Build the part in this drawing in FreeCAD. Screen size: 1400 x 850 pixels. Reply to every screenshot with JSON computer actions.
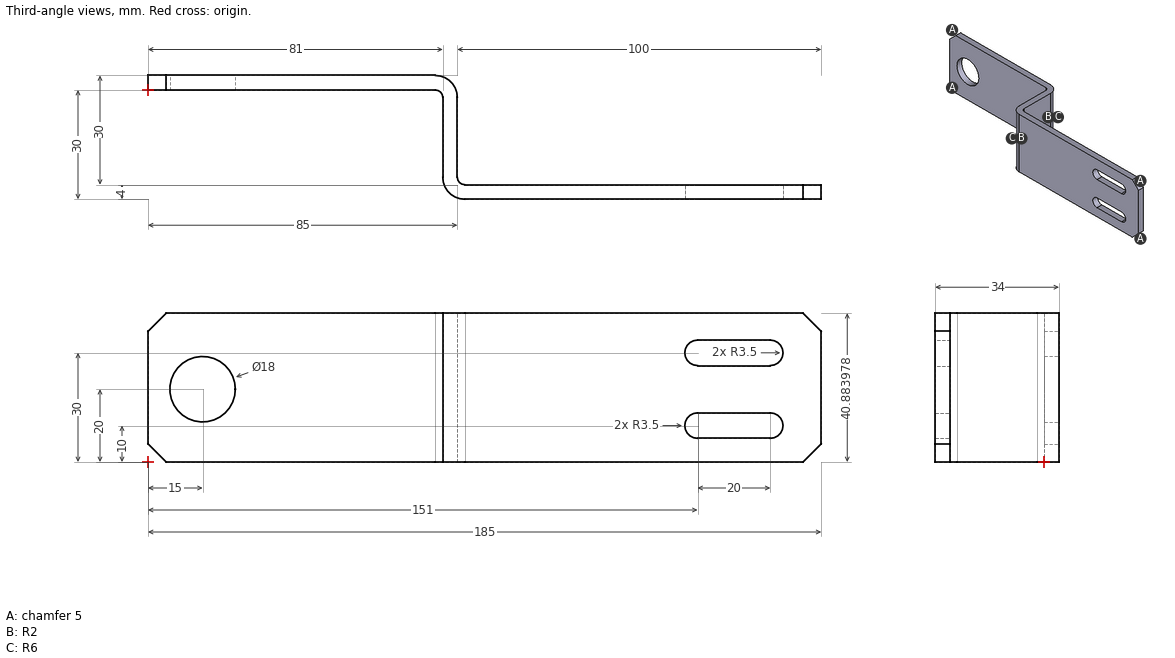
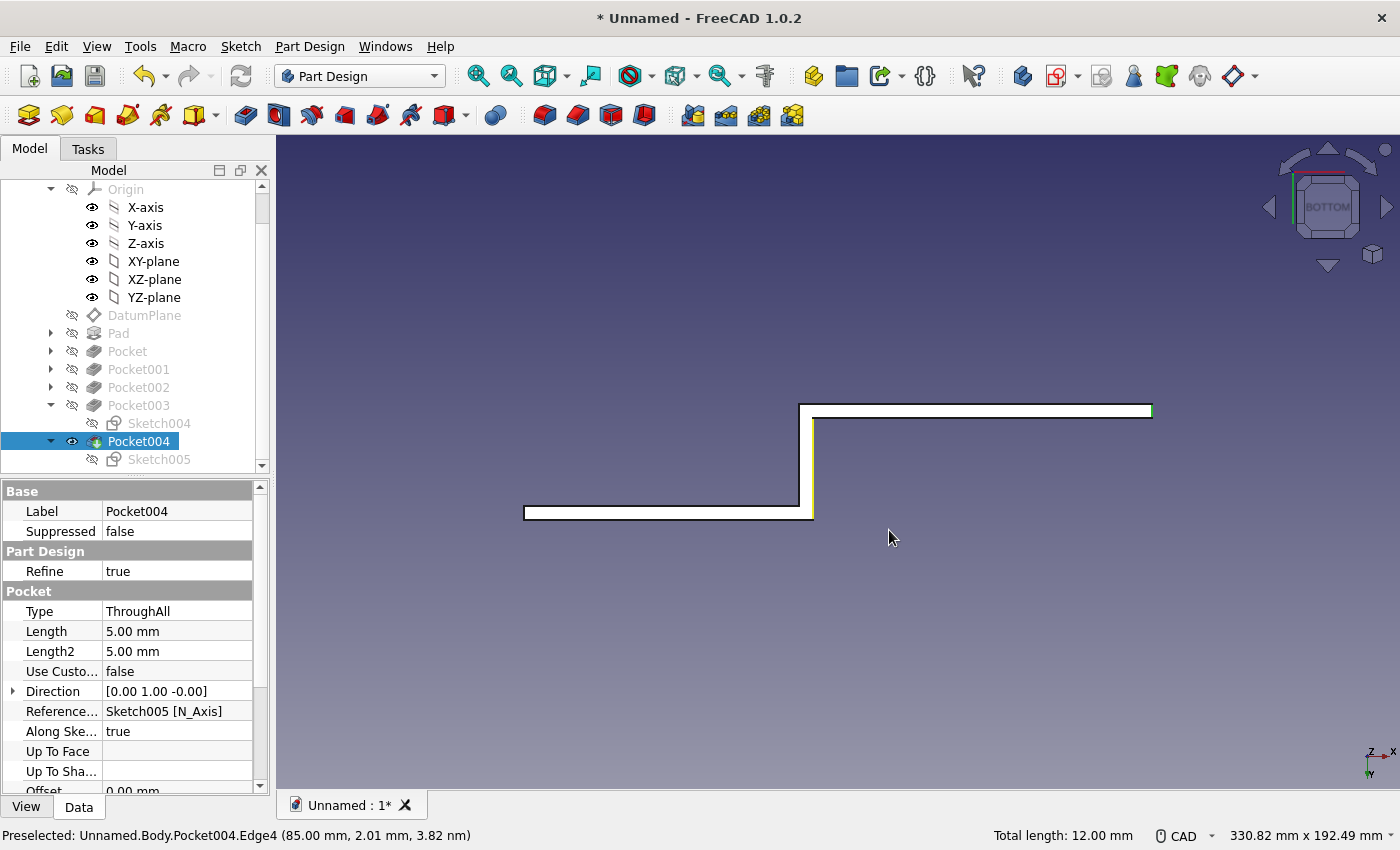
{"action": "scroll", "coordinate": [524, 512], "scroll_direction": "up", "scroll_amount": 6}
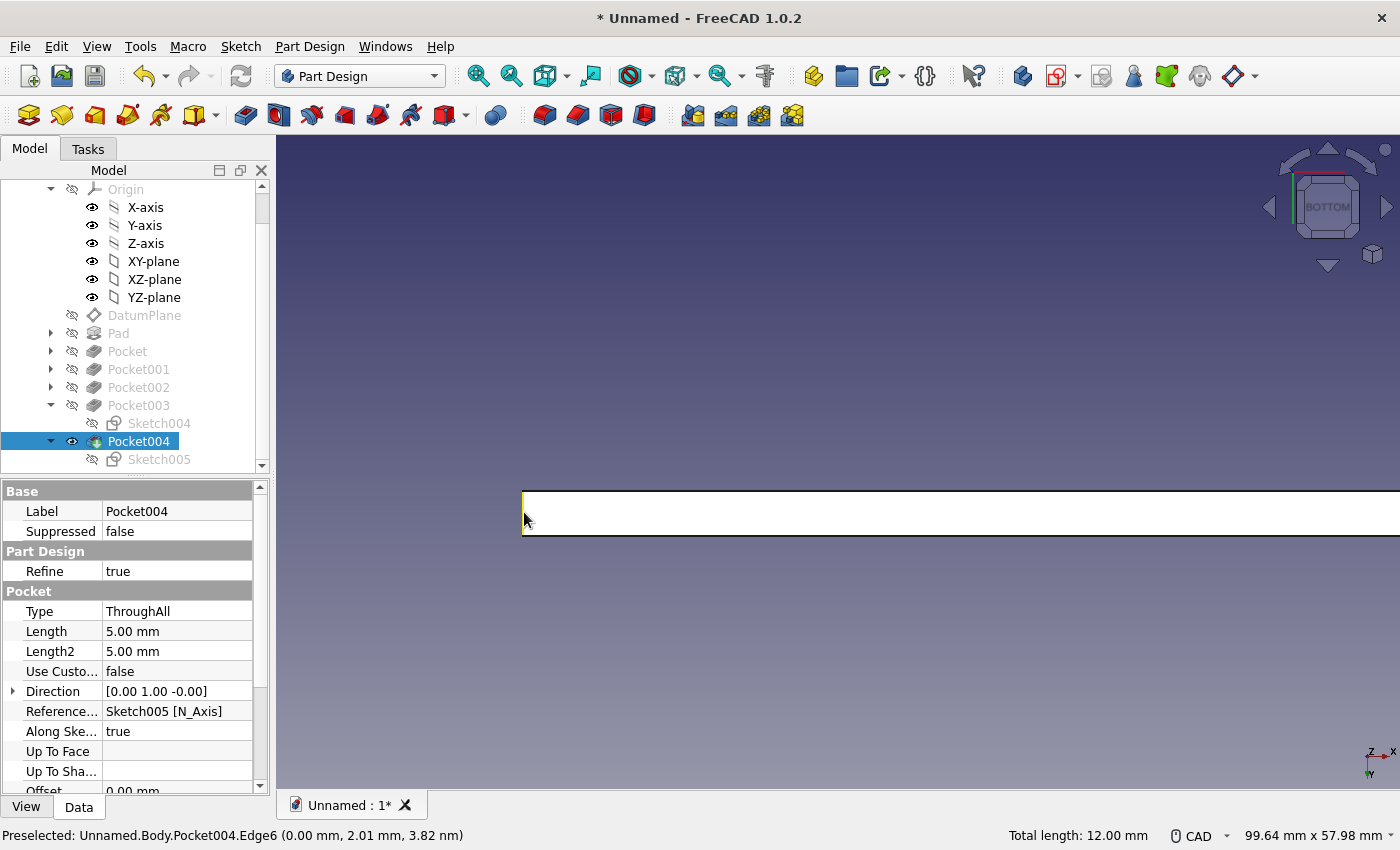
{"action": "left_click", "coordinate": [479, 76]}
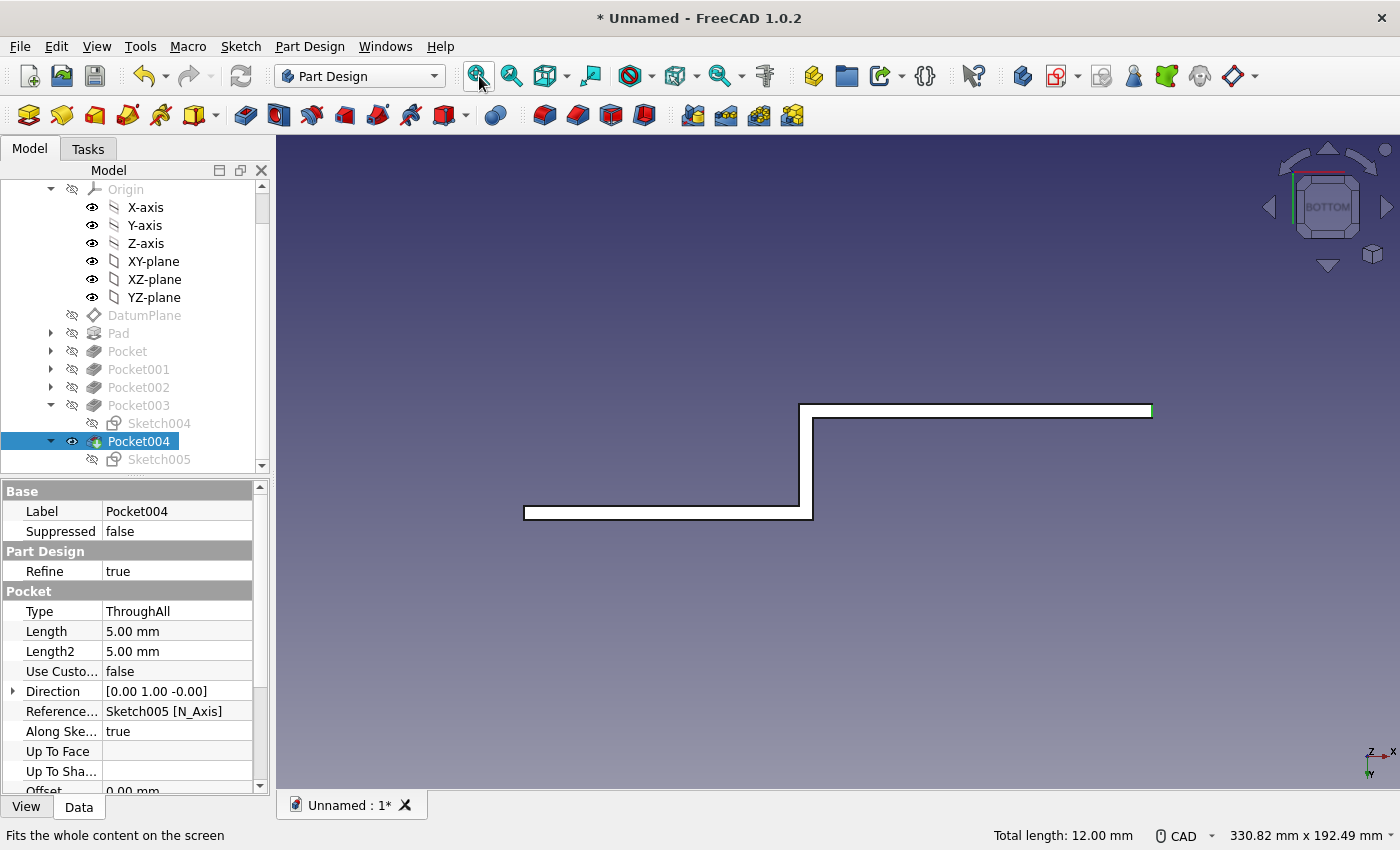
{"action": "key", "text": "4"}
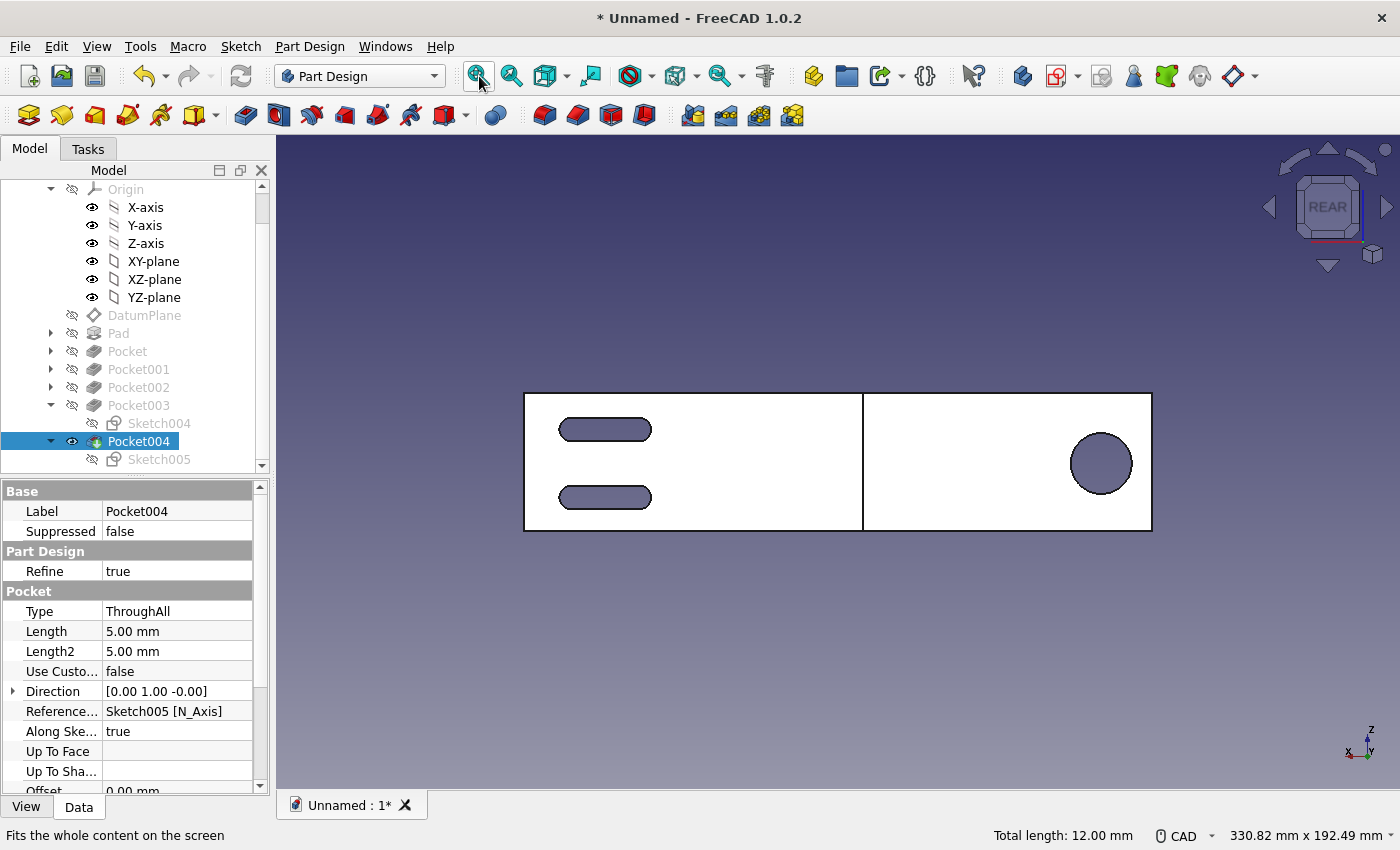
{"action": "scroll", "coordinate": [1152, 530], "scroll_direction": "up", "scroll_amount": 6}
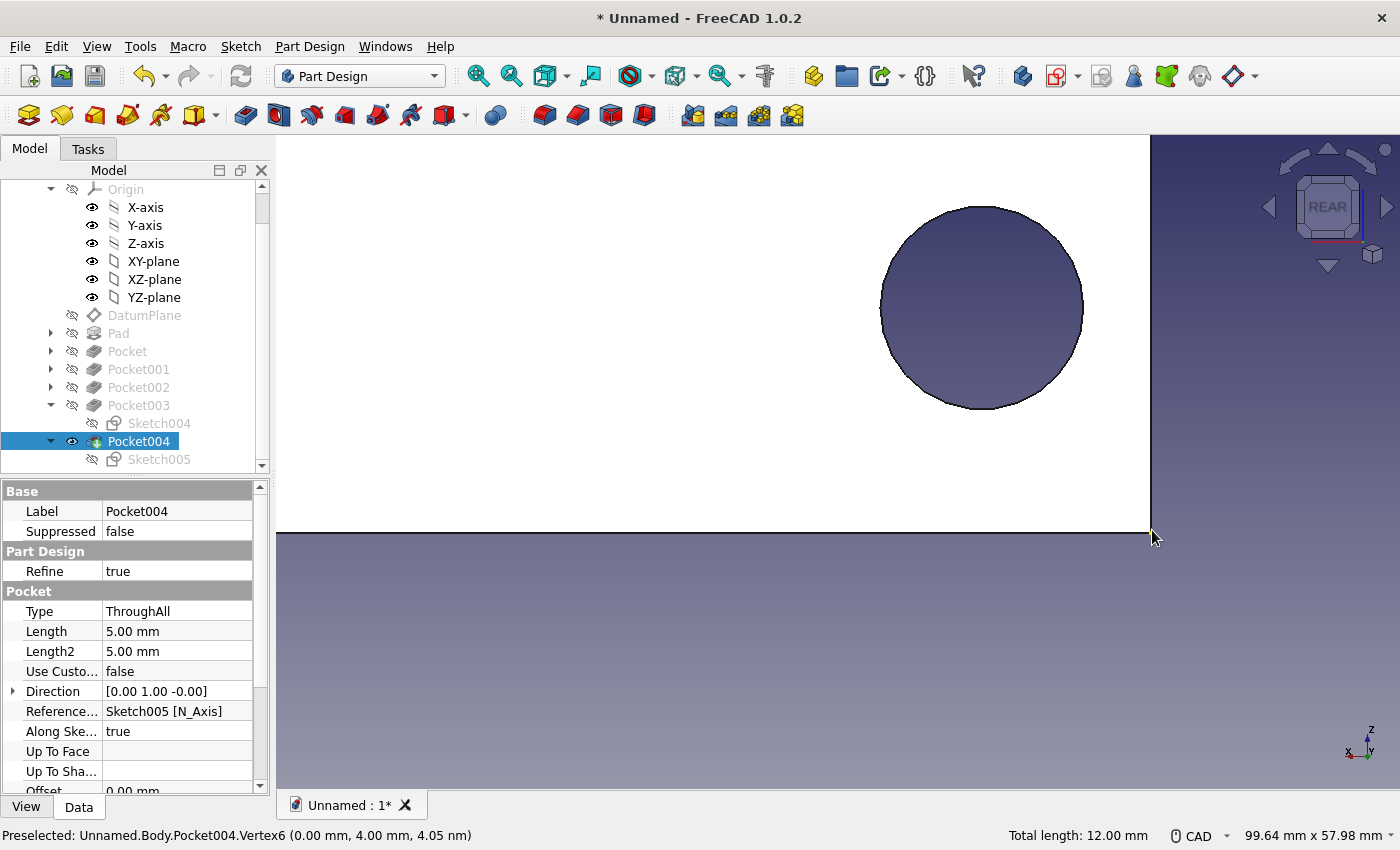
{"action": "key", "text": "v f"}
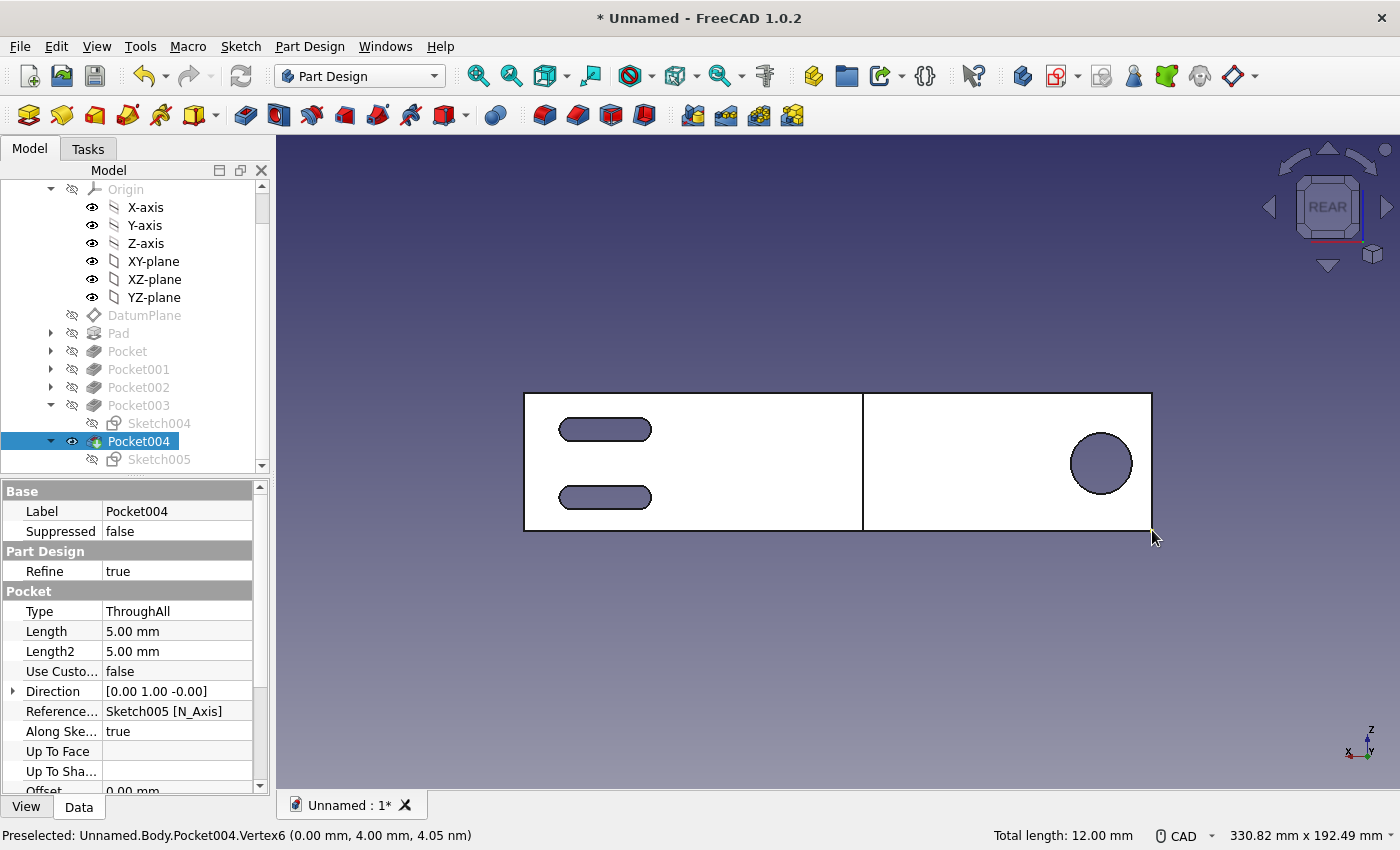
{"action": "key", "text": "6"}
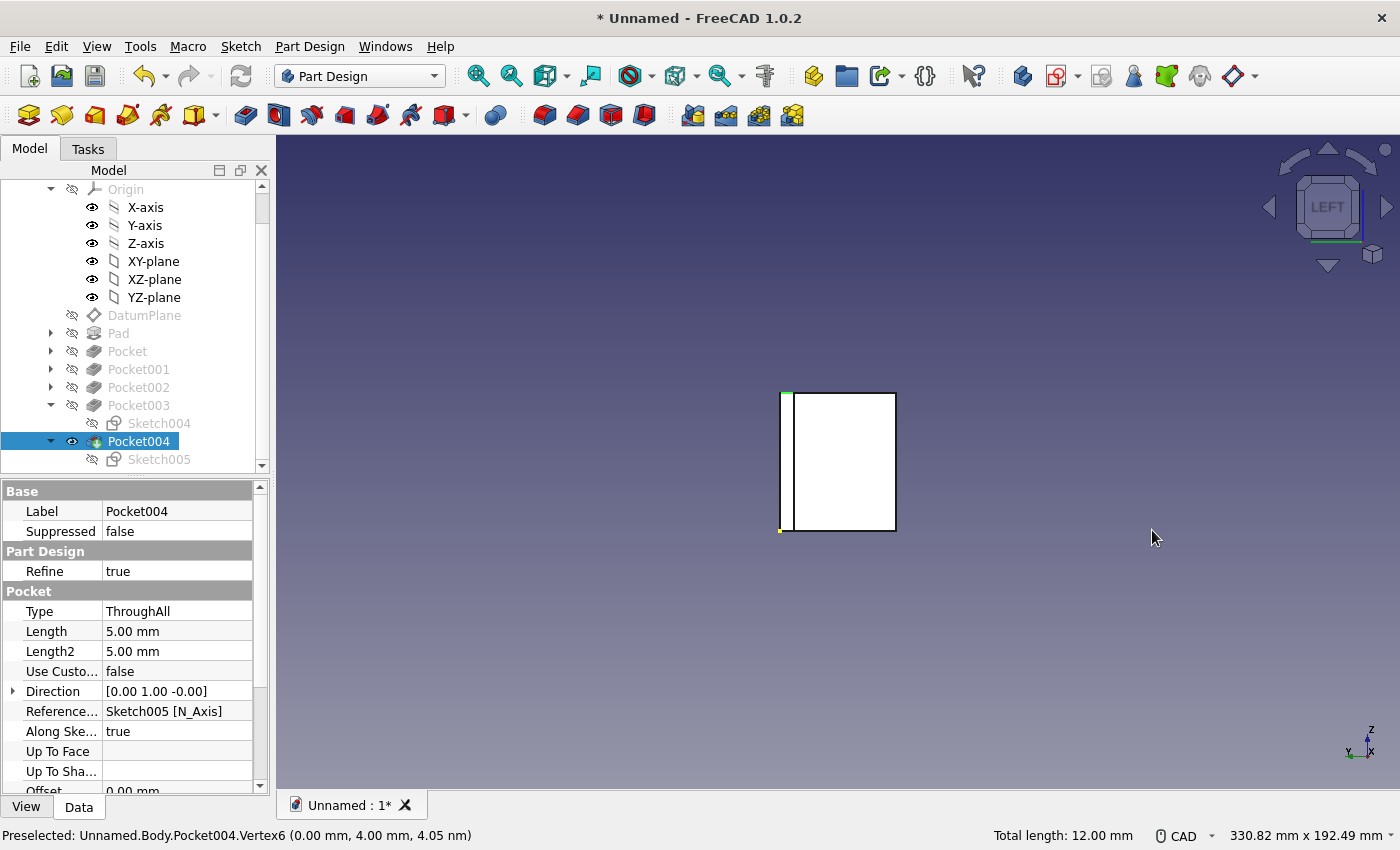
{"action": "key", "text": "v f"}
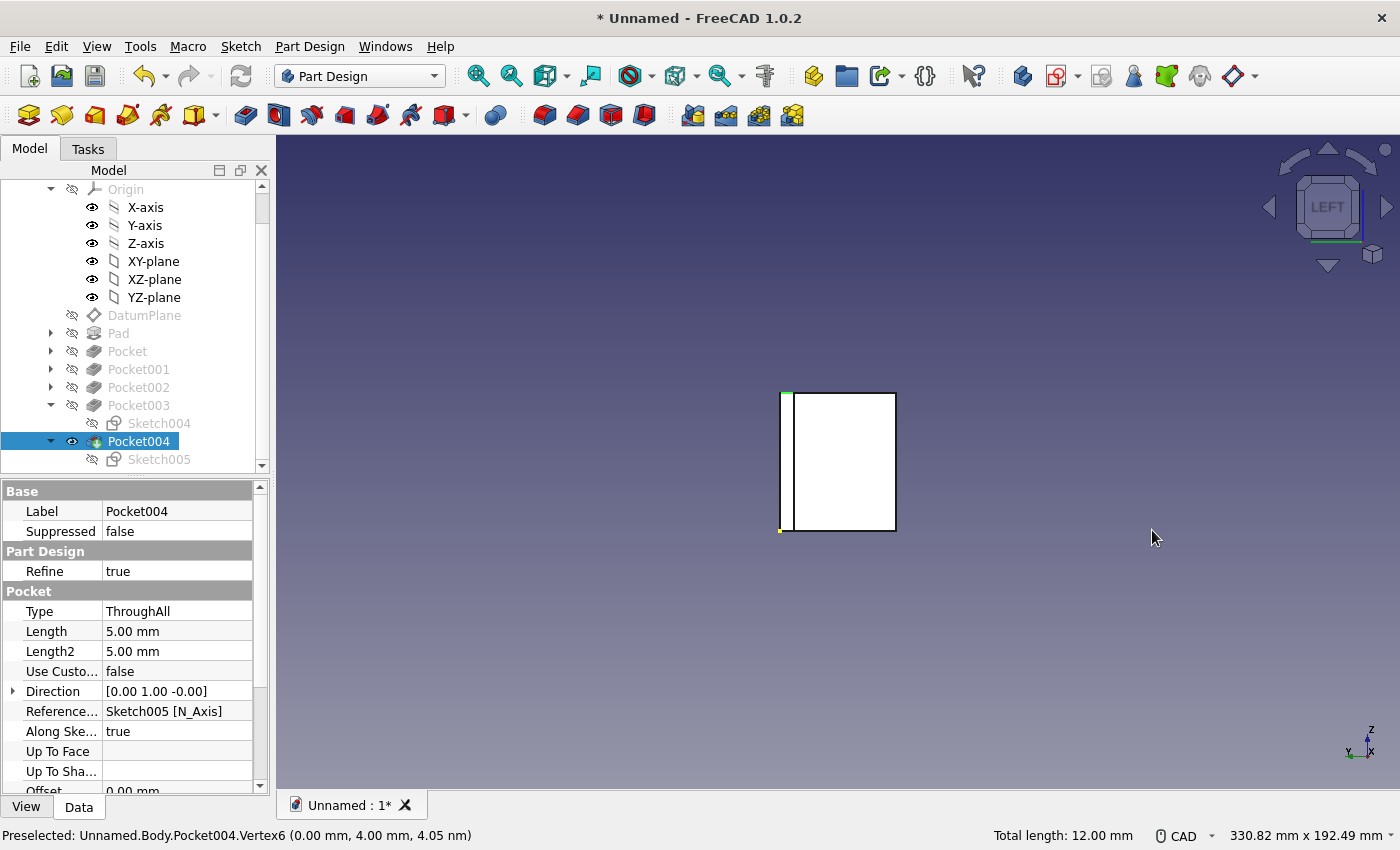
{"action": "left_click", "coordinate": [787, 530], "text": "ctrl"}